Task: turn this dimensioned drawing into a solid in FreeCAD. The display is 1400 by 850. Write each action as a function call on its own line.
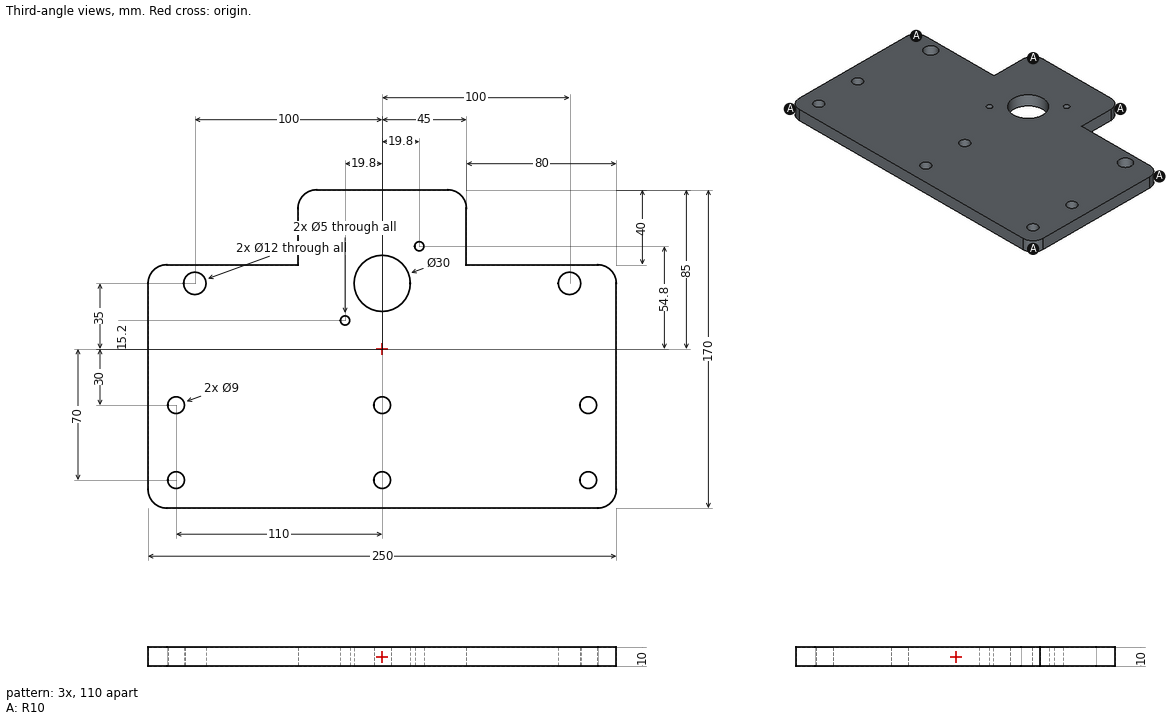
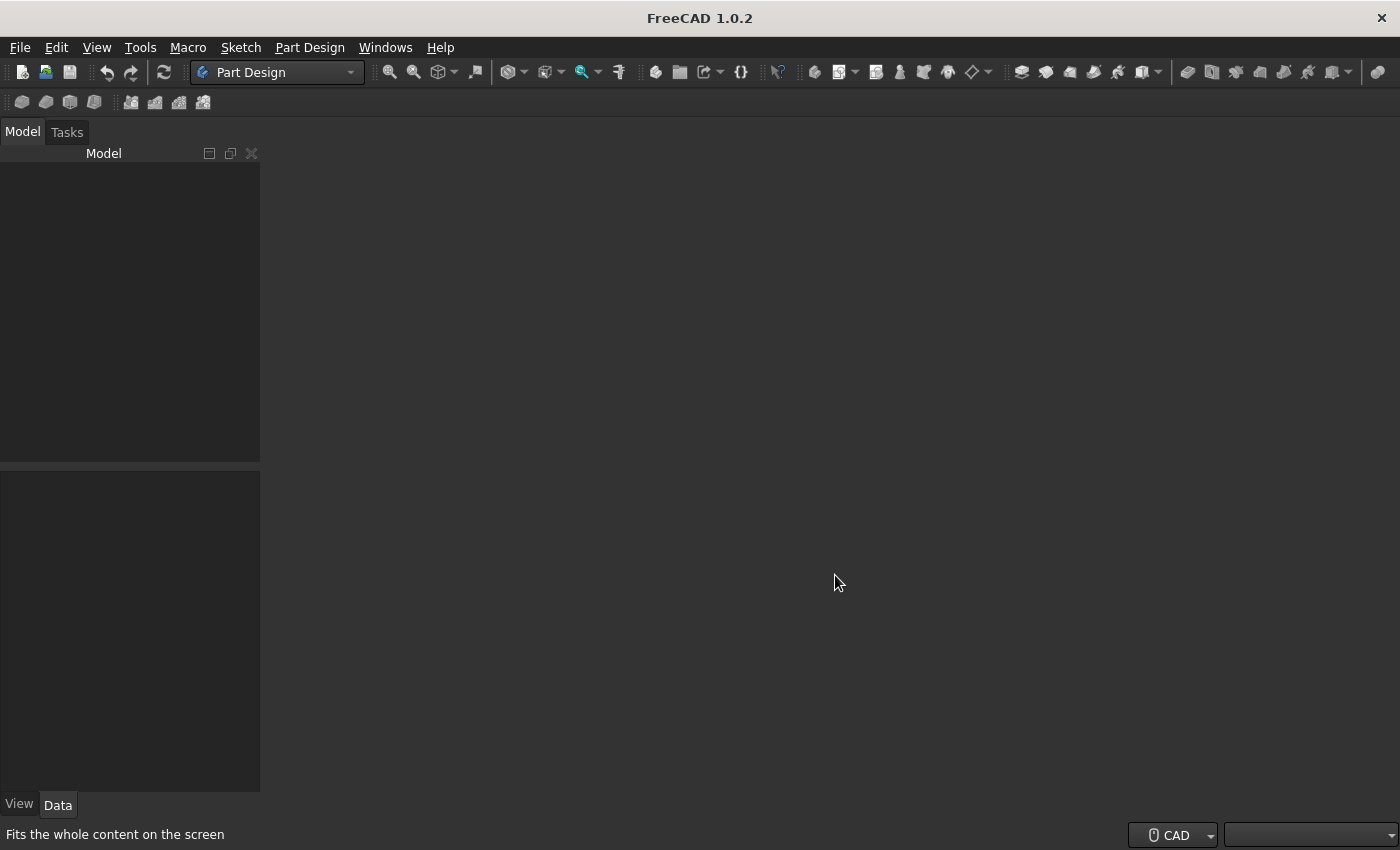
click(22, 72)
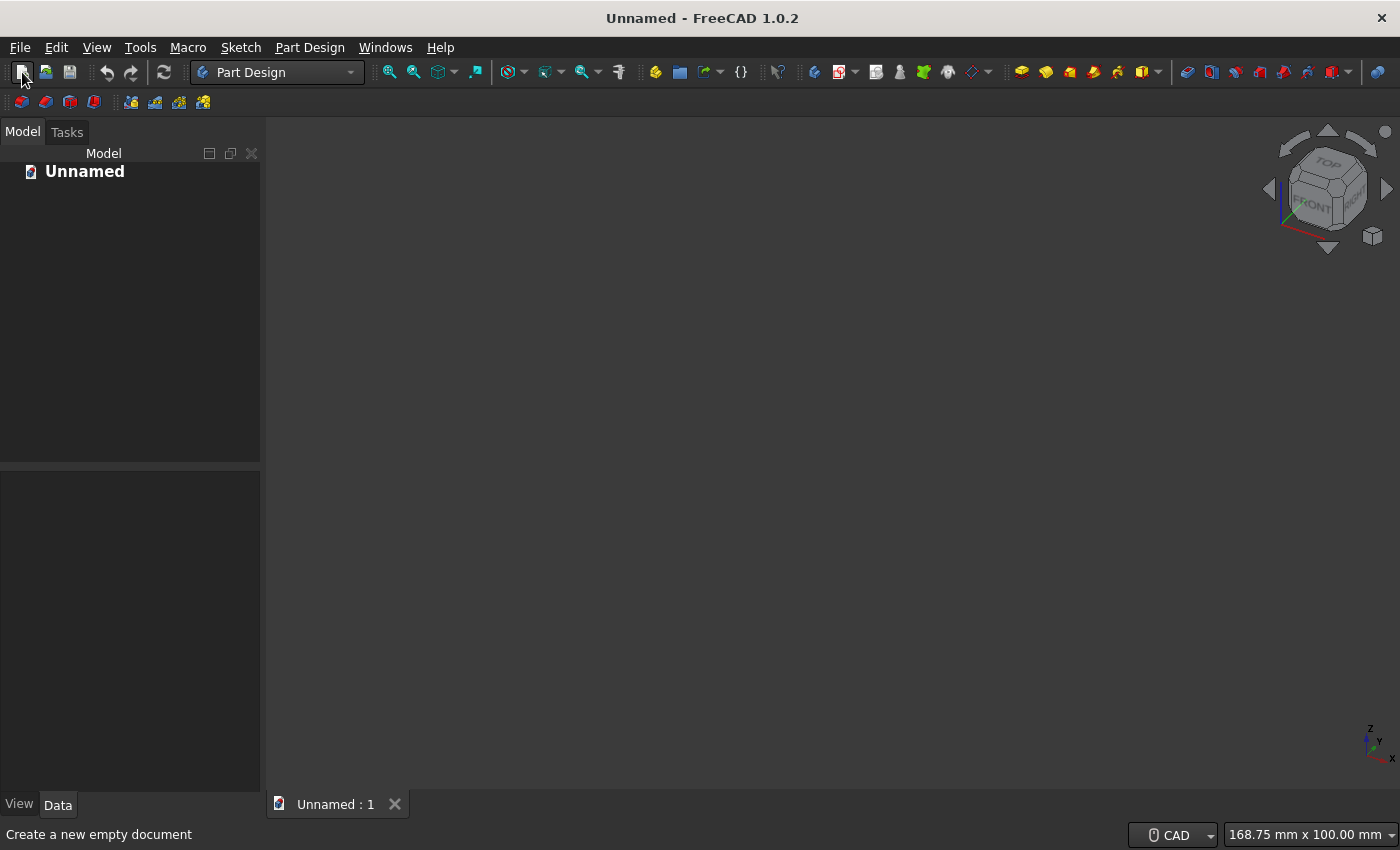
click(840, 72)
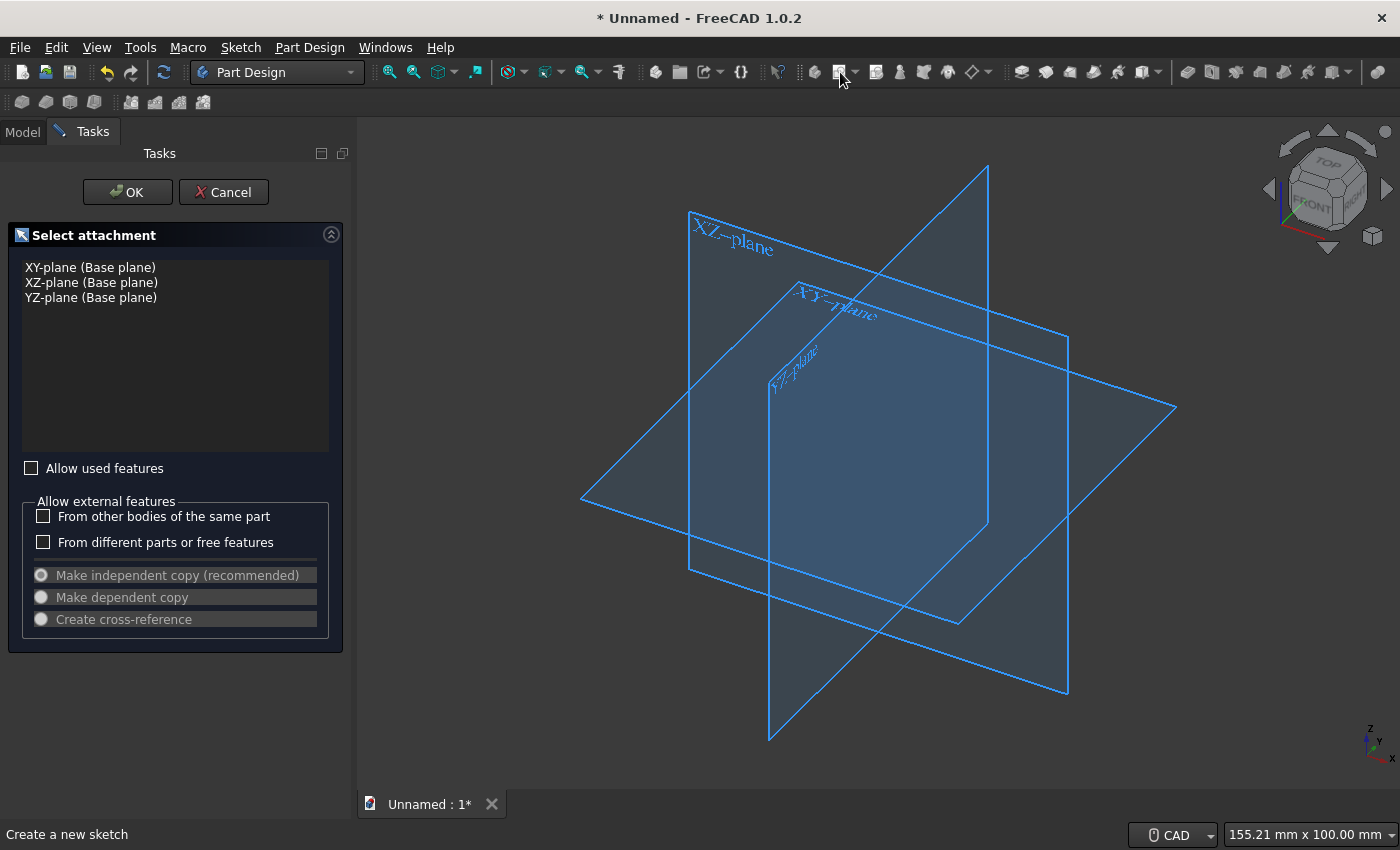
click(82, 268)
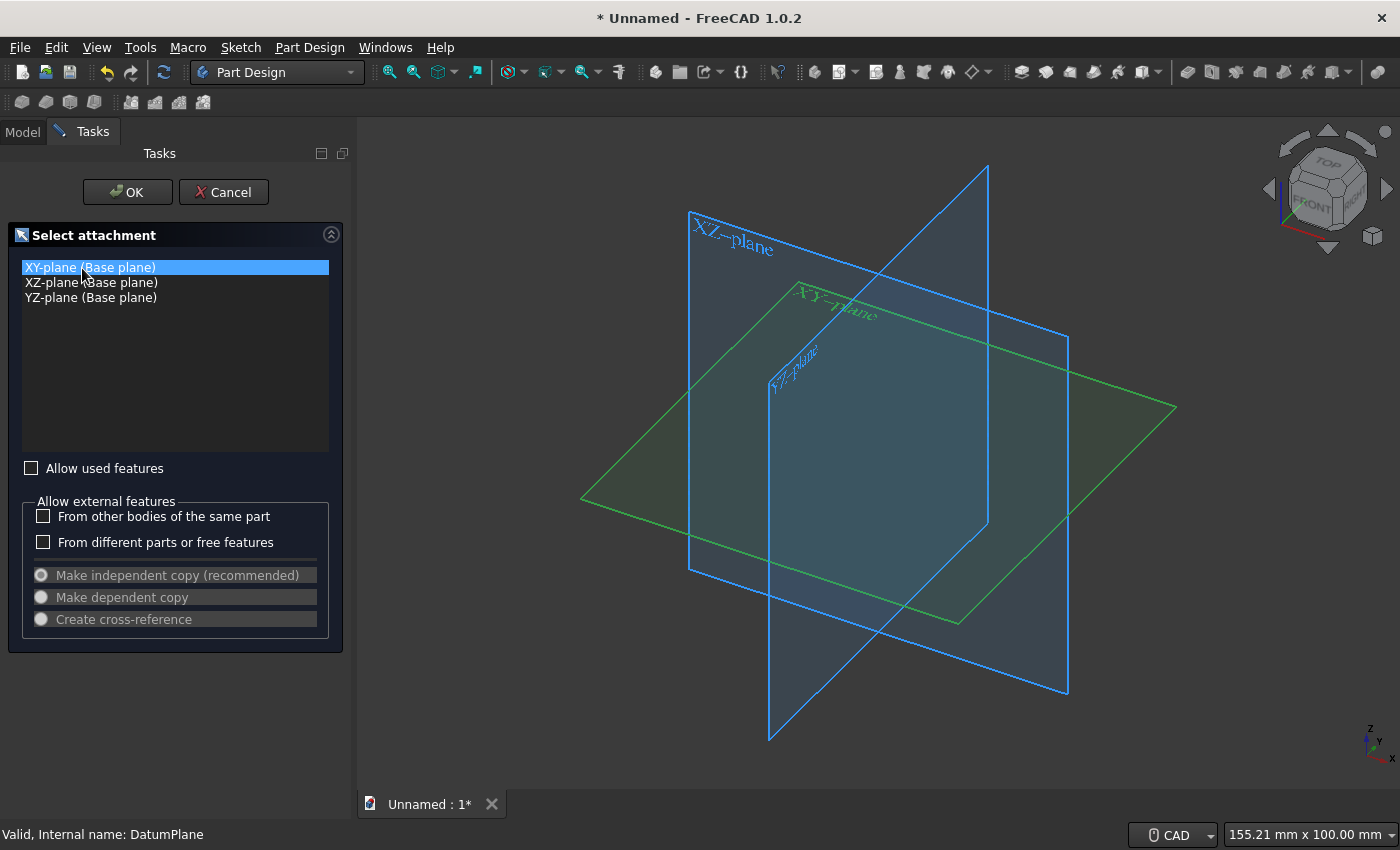
click(128, 192)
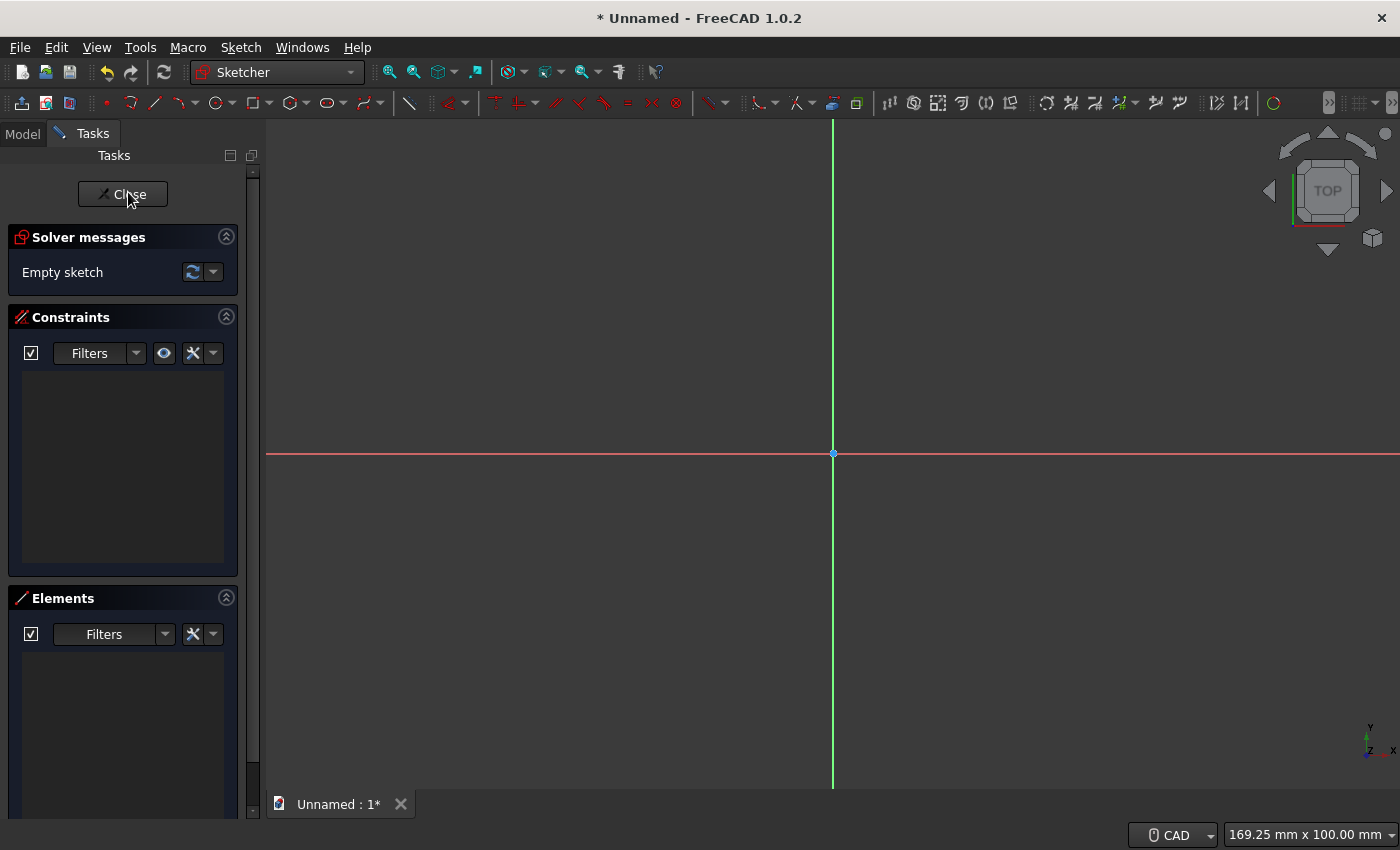
scroll(725, 454, down, 5)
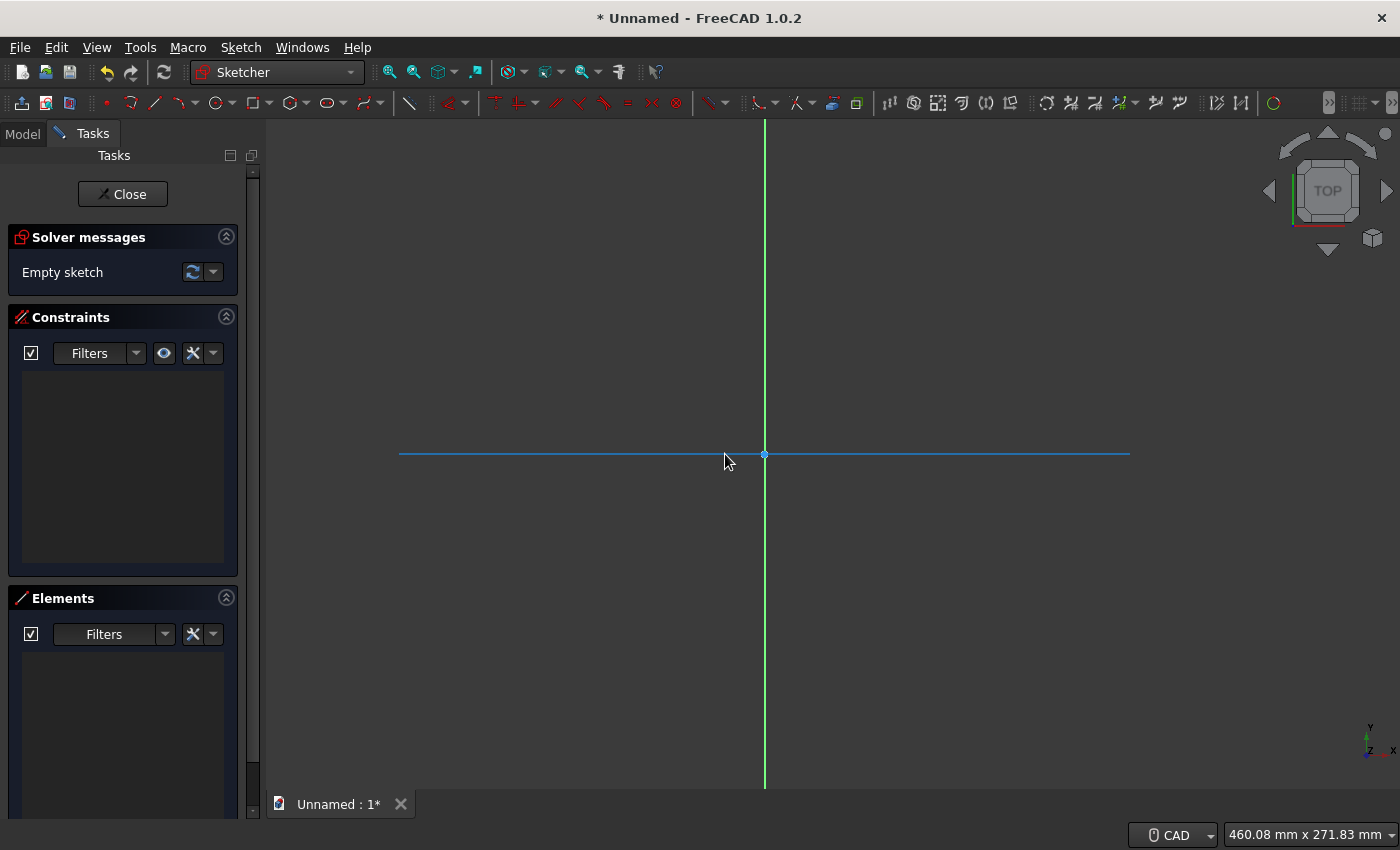
click(272, 104)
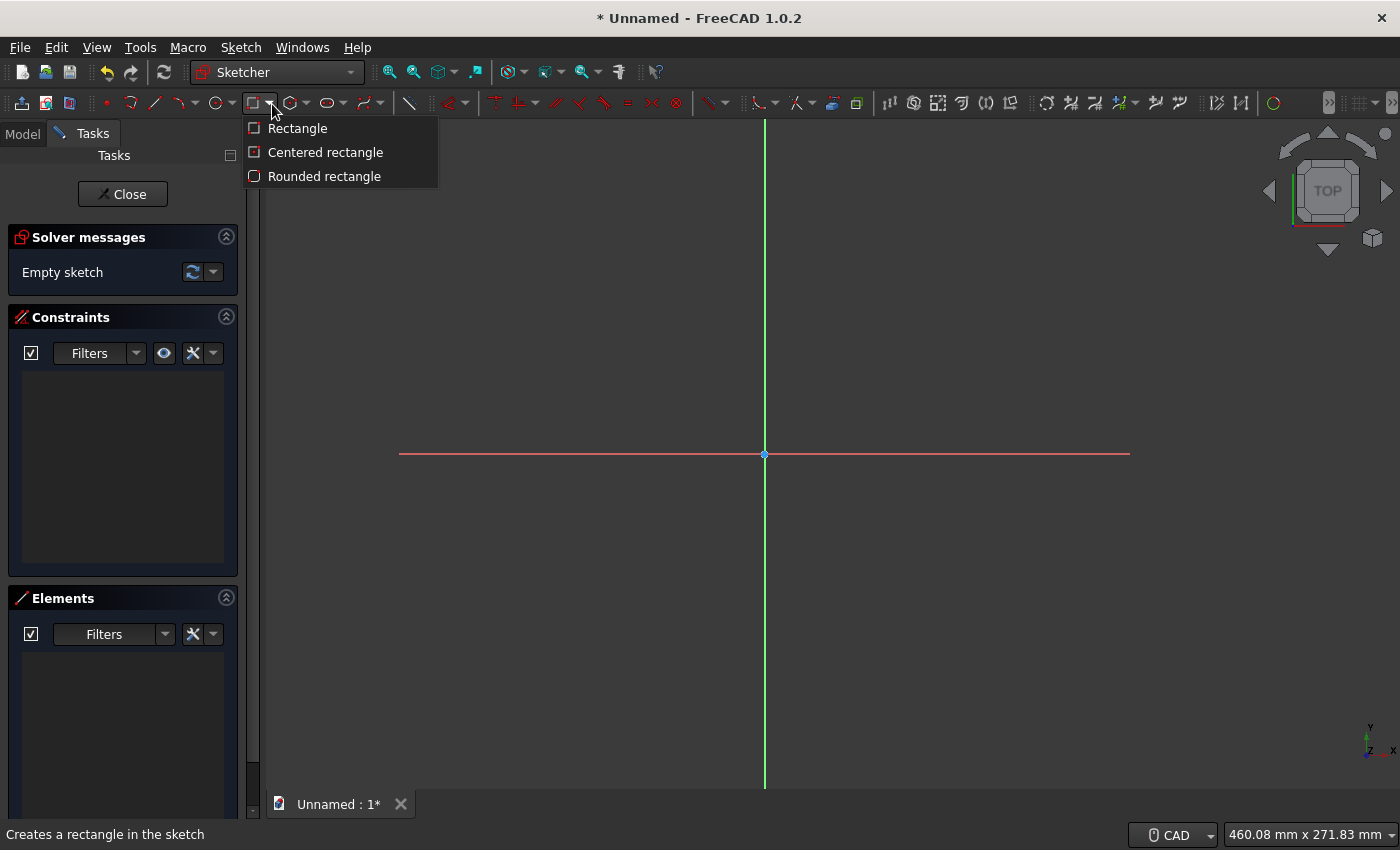
click(340, 152)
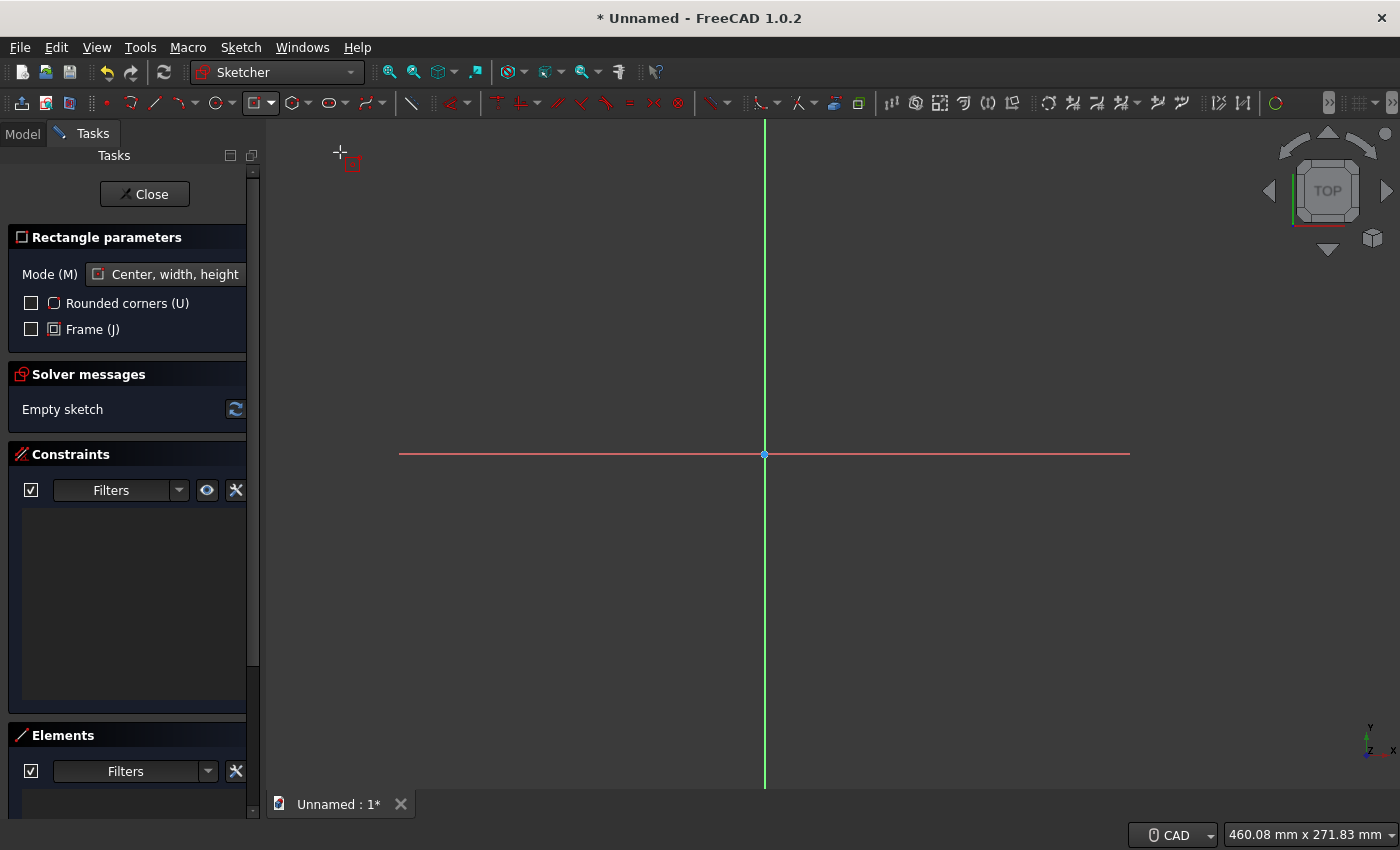
click(765, 454)
move(1073, 245)